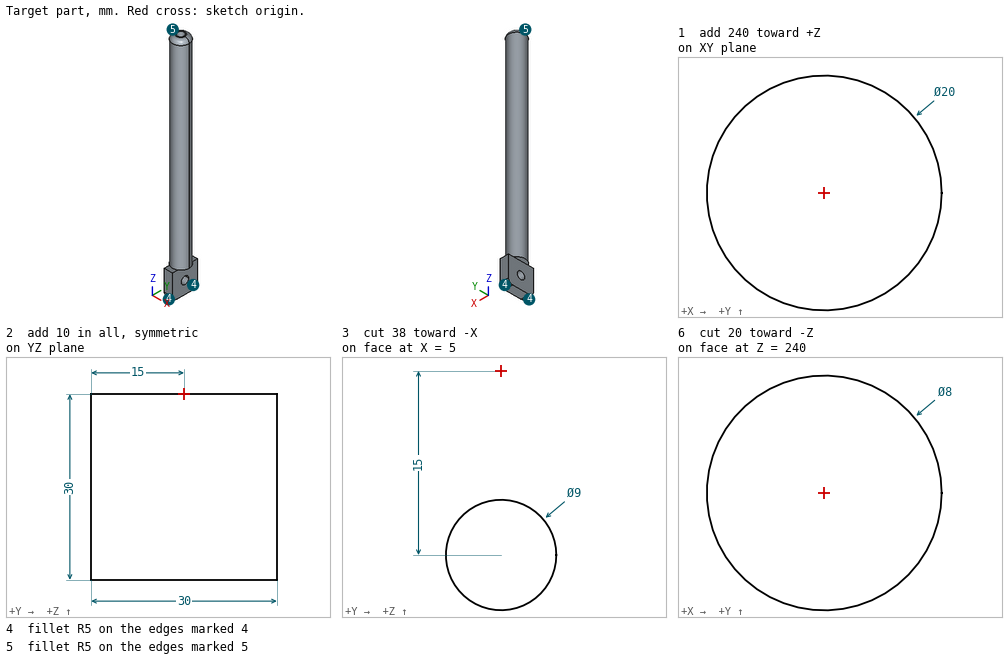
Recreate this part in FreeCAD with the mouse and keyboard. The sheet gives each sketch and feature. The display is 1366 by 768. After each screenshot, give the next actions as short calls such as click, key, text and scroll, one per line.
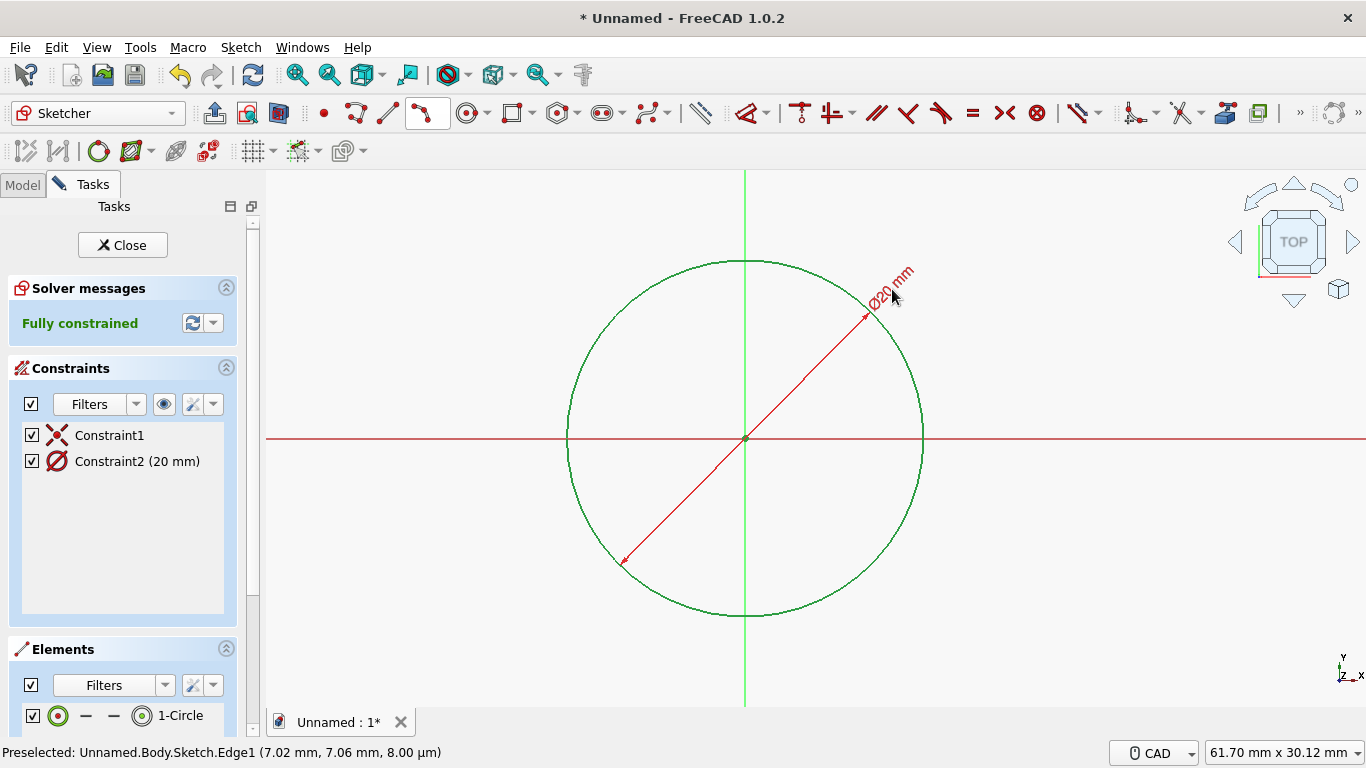
click(123, 245)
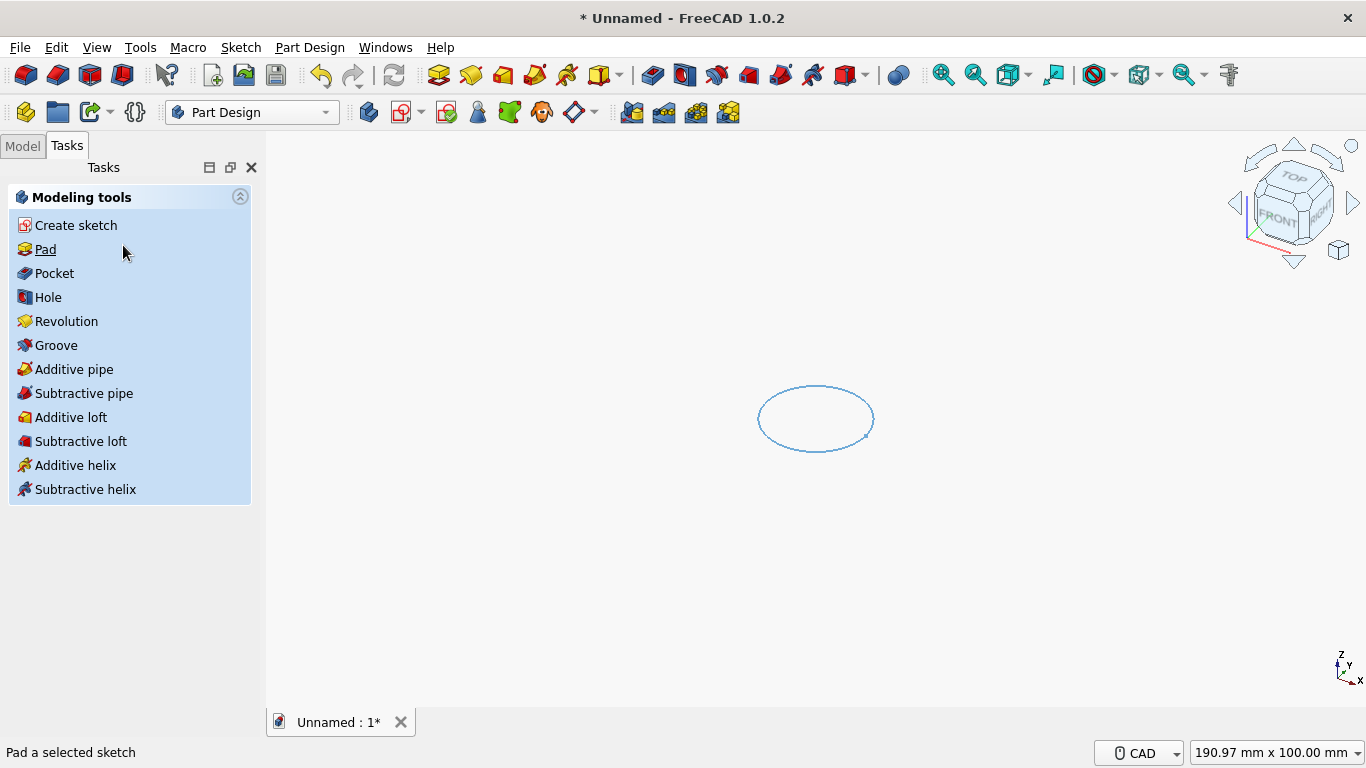
click(440, 76)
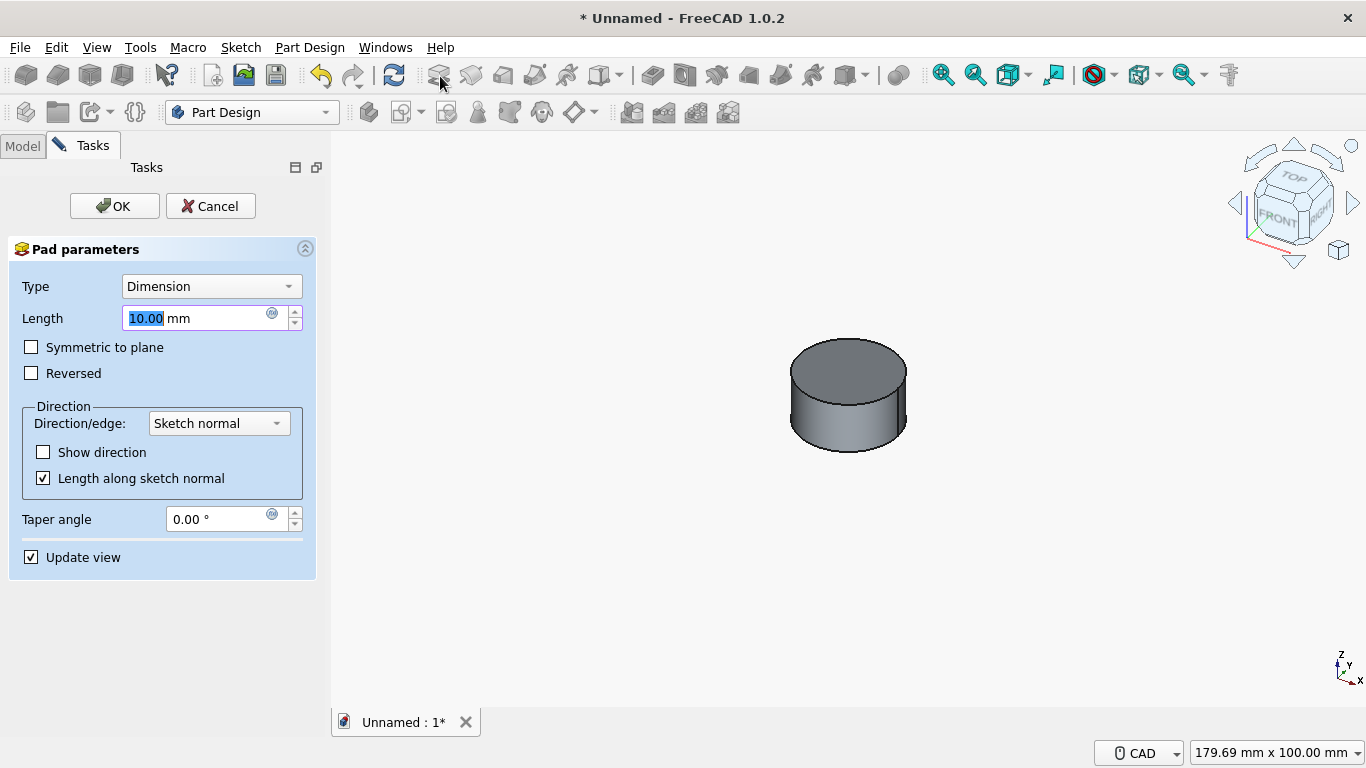
text(240)
key(Tab)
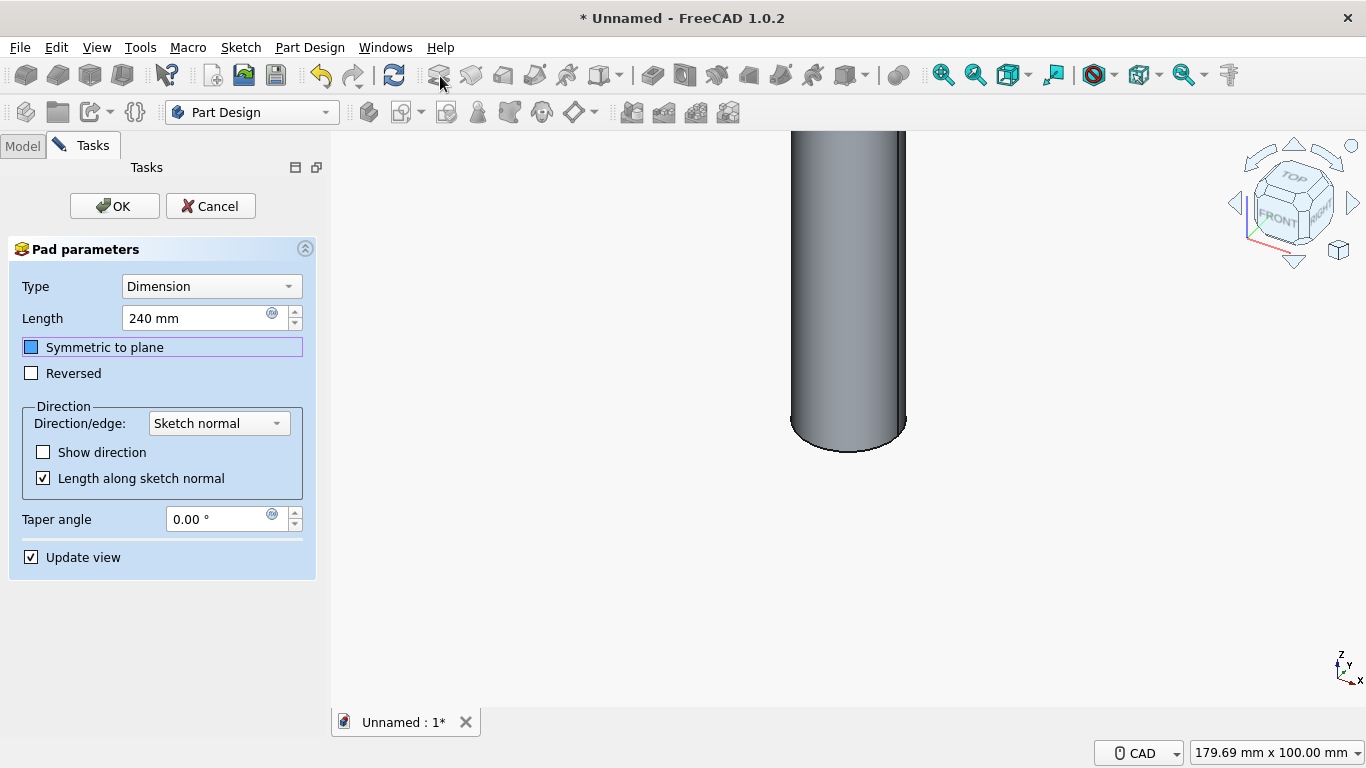
click(115, 206)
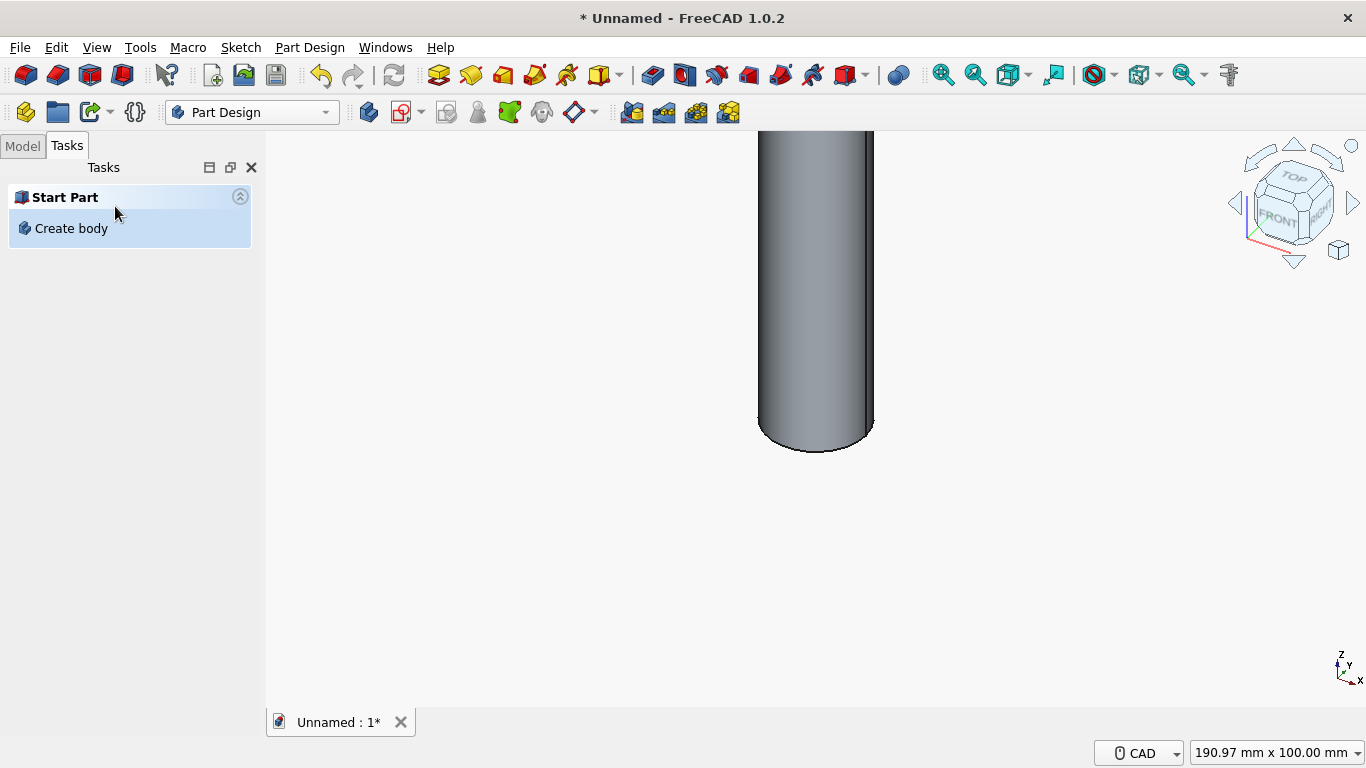
key(v)
key(f)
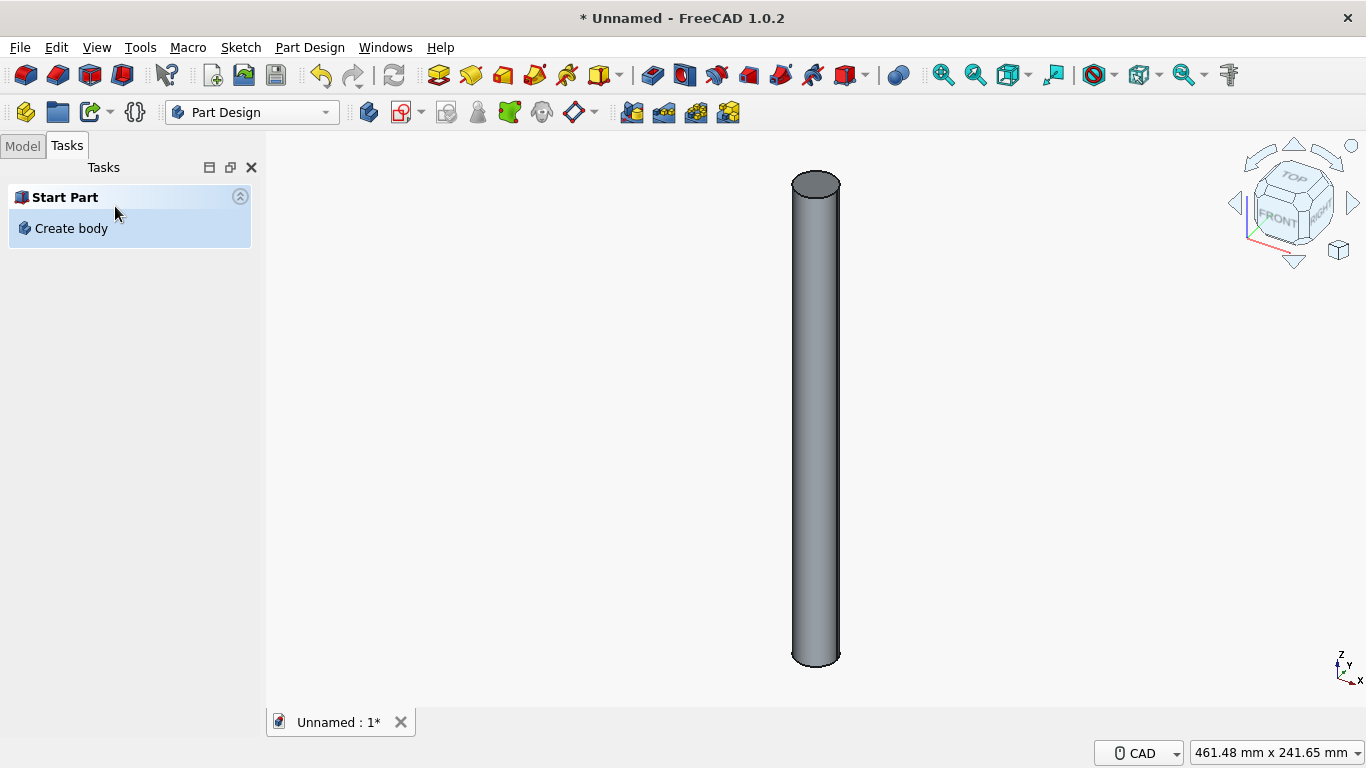
click(402, 112)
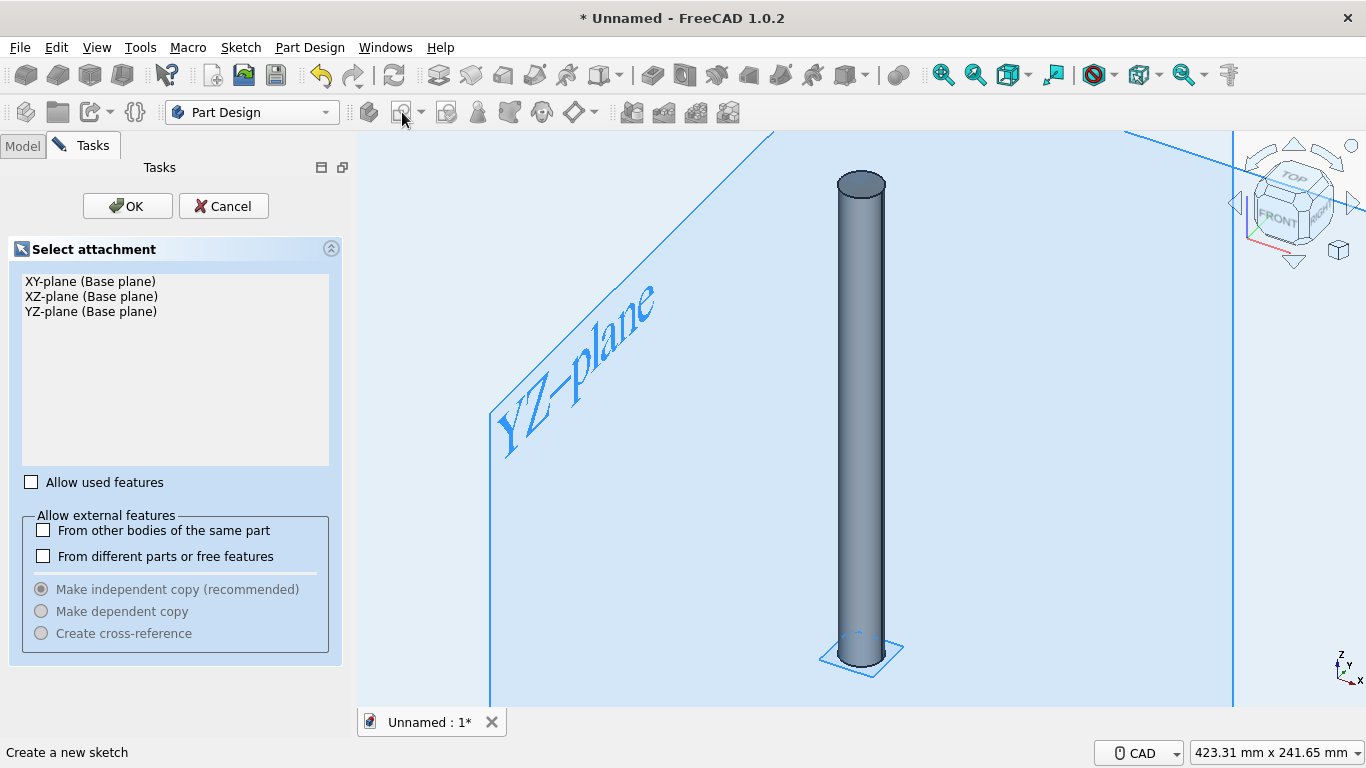
click(82, 312)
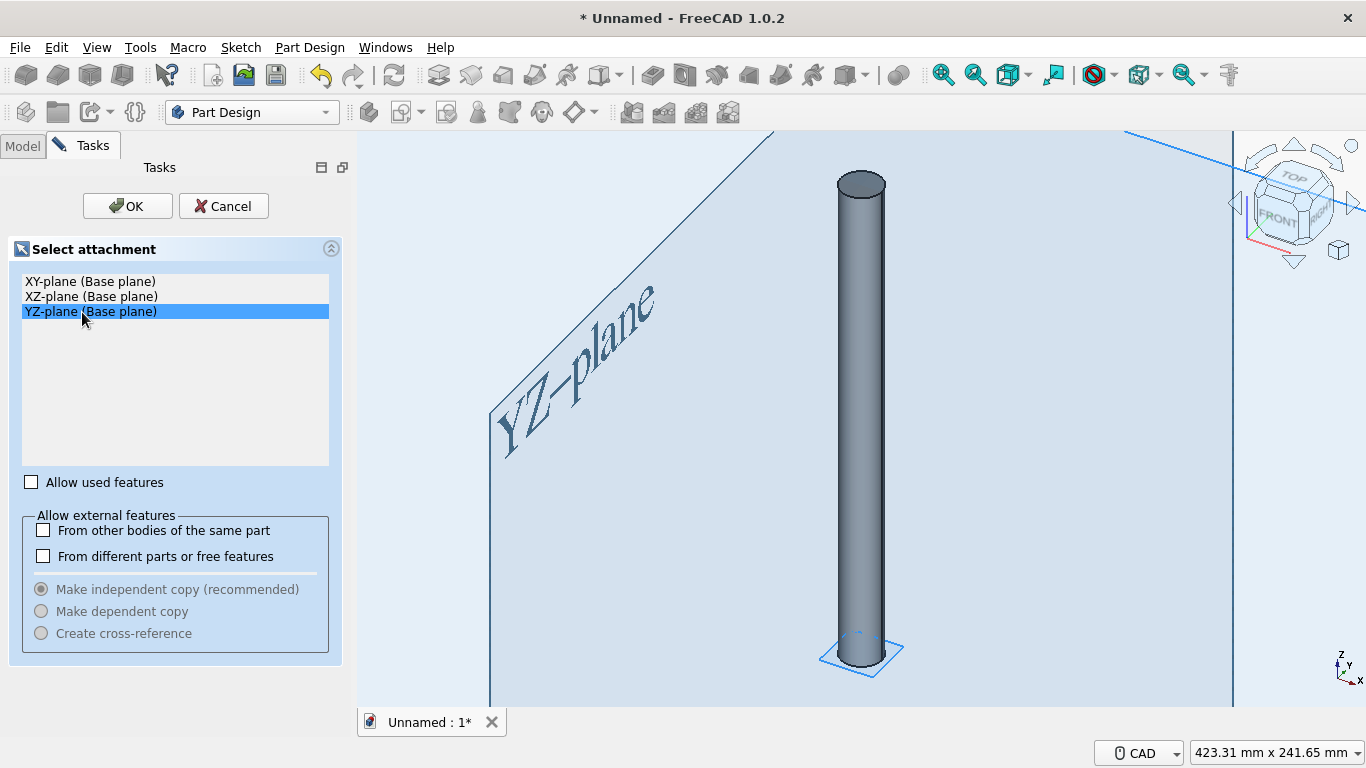
click(128, 206)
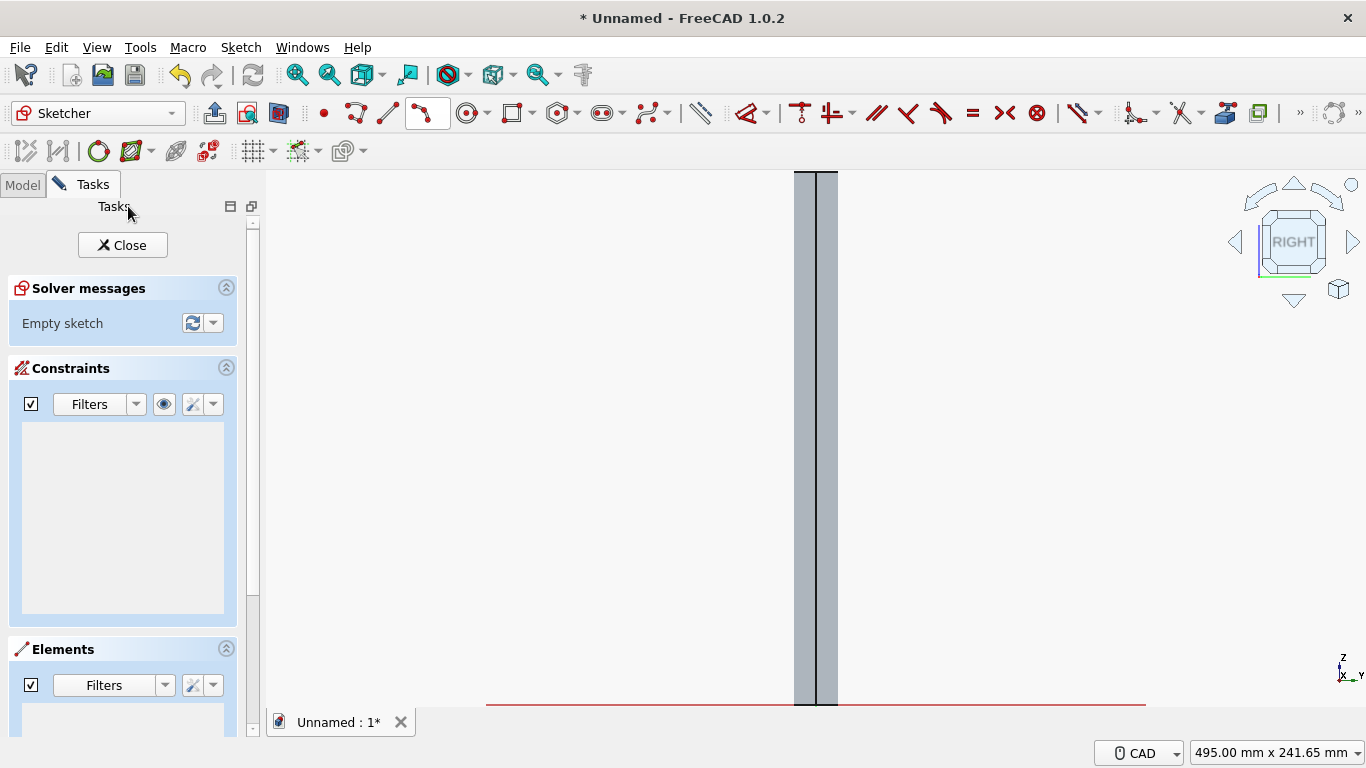
click(280, 114)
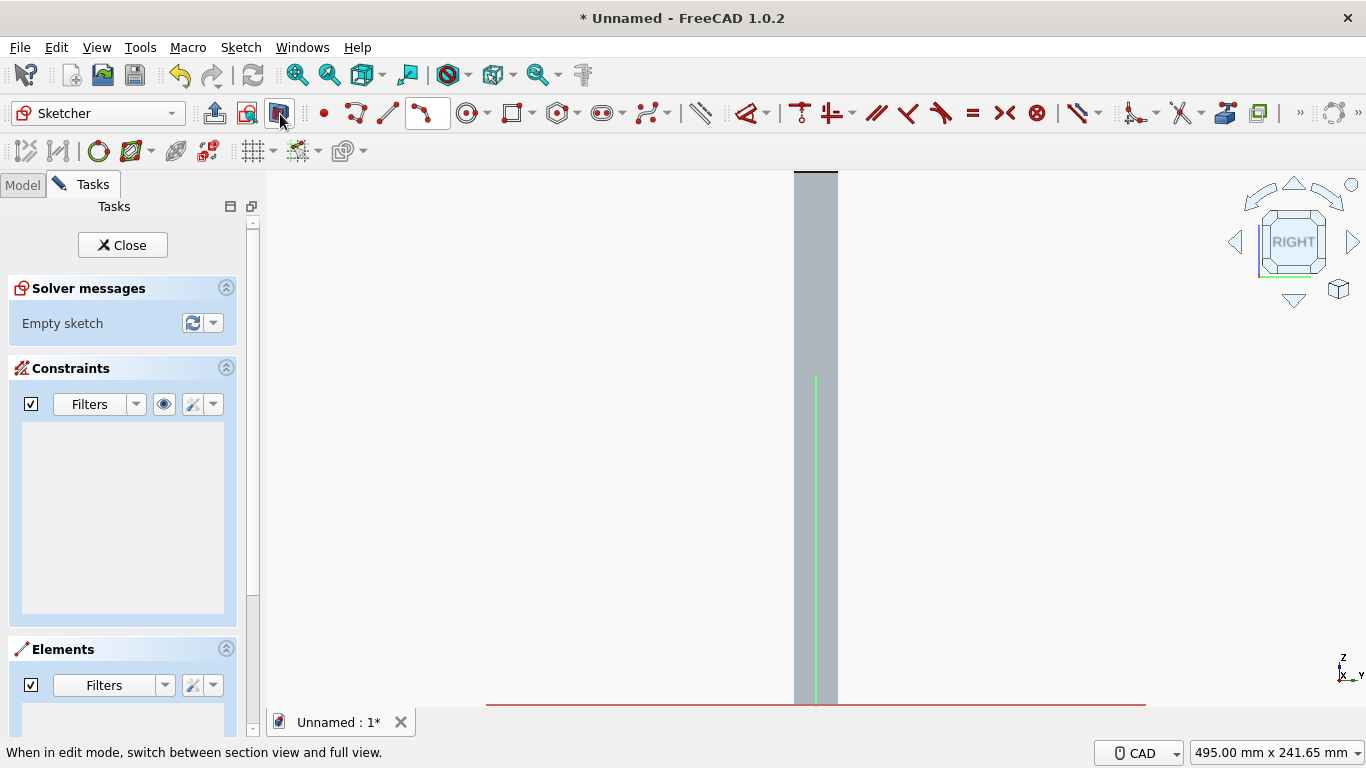
scroll(748, 438, down, 5)